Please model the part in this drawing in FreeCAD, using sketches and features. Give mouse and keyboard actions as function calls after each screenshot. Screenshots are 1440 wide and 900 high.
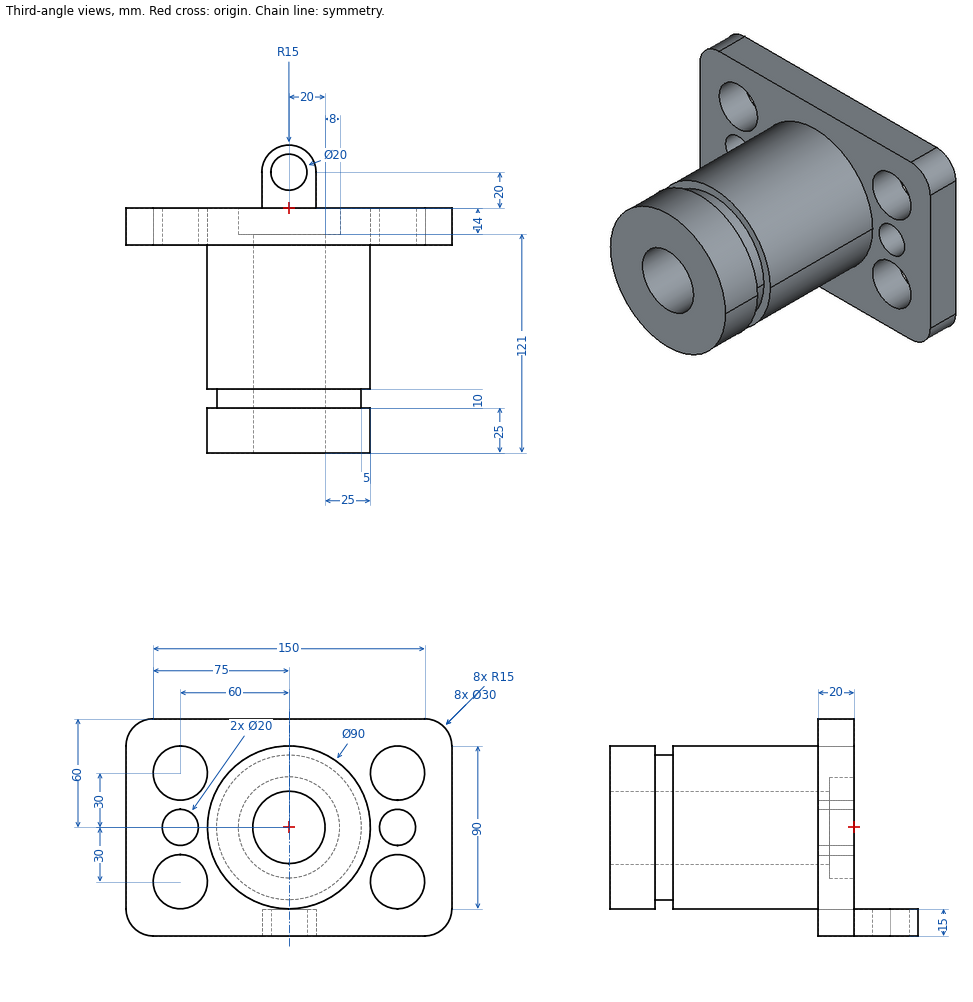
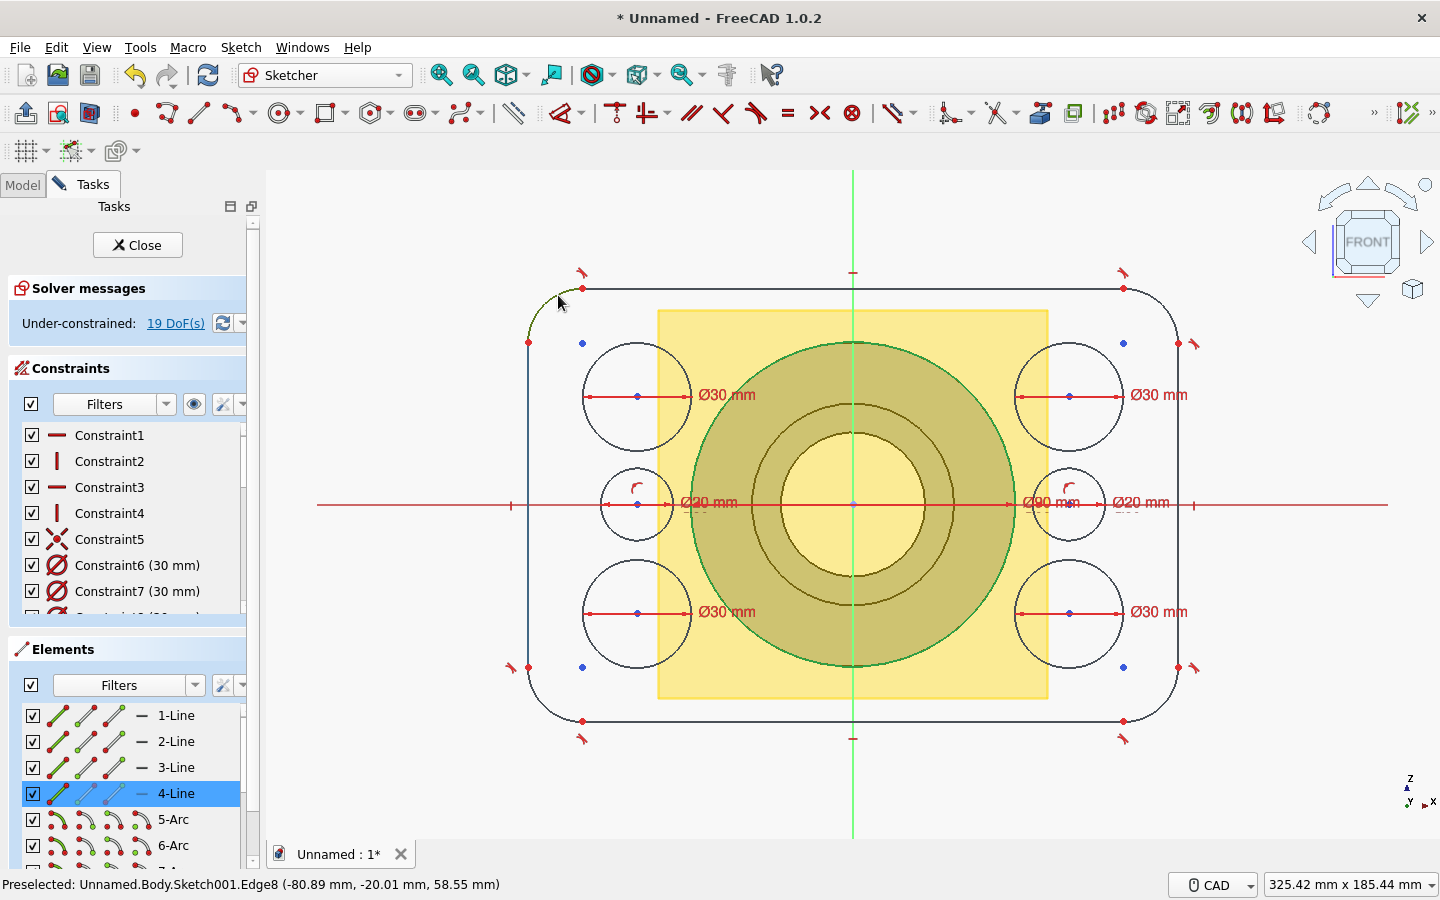
click(756, 114)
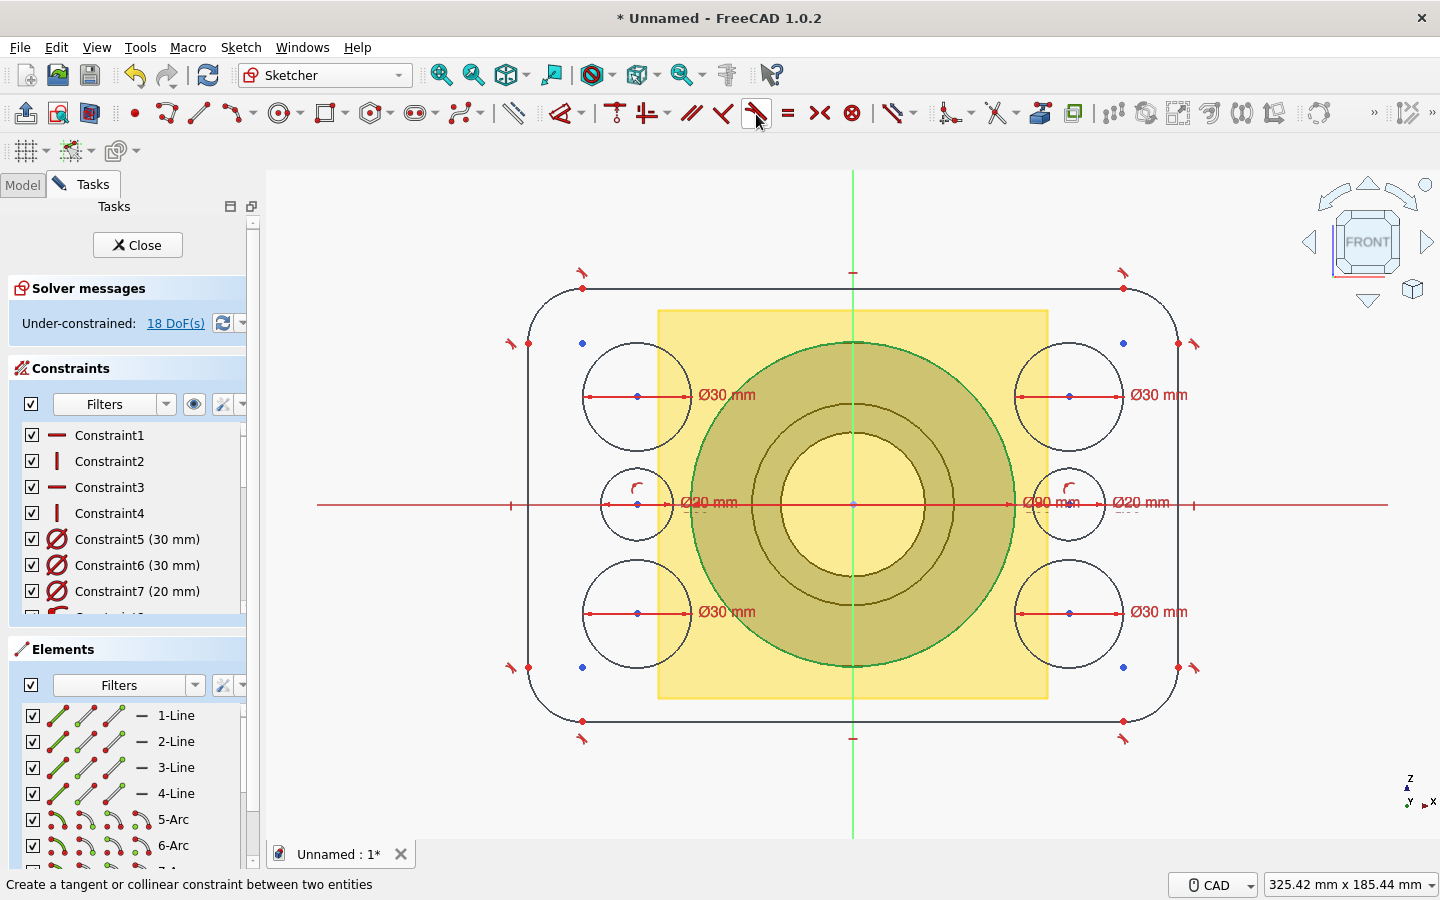
click(1172, 319)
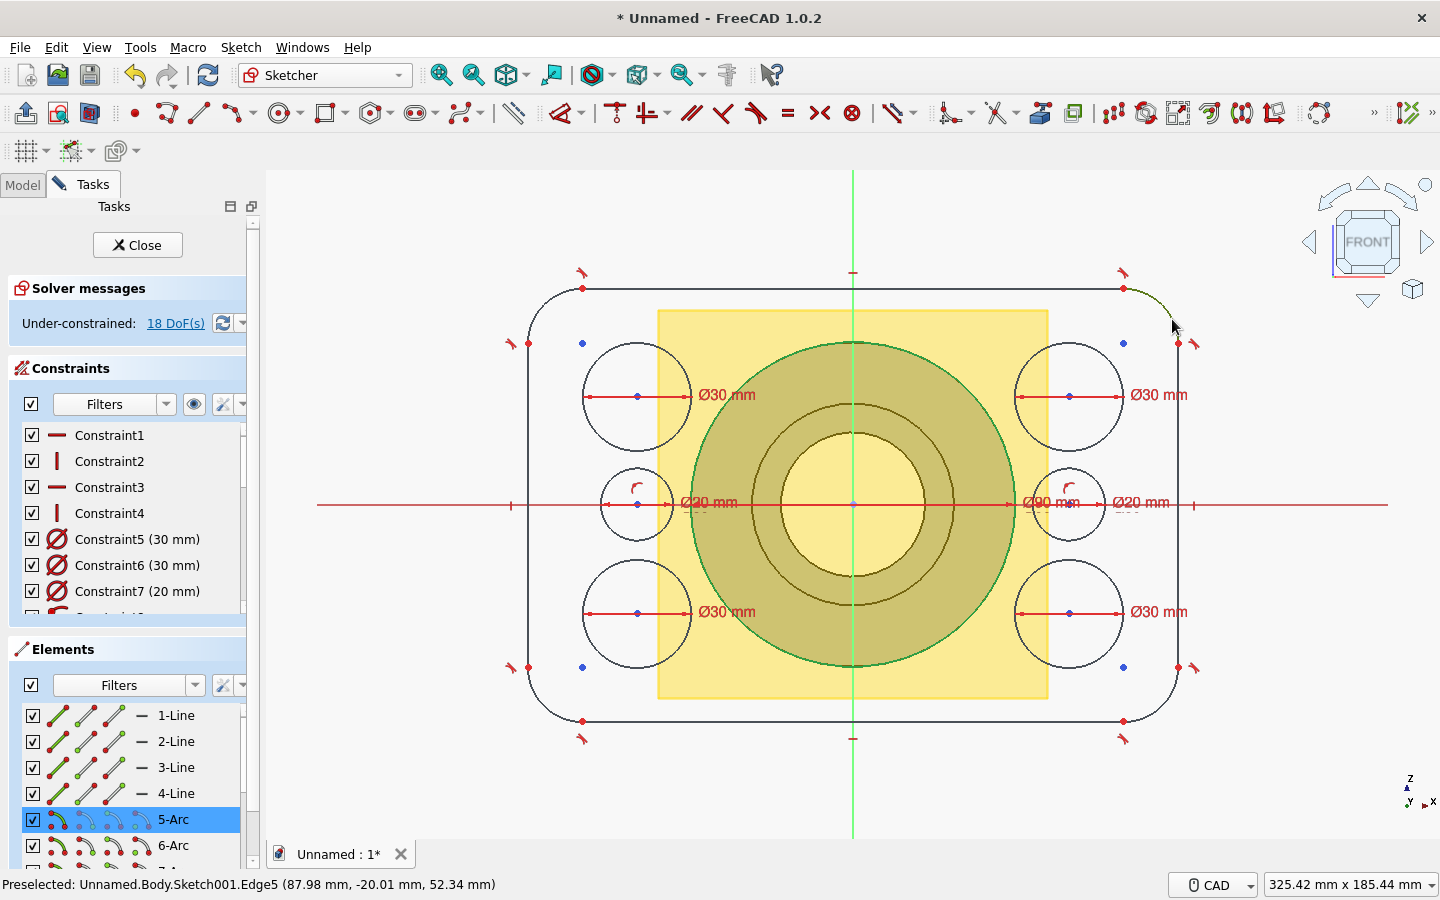
click(1148, 716)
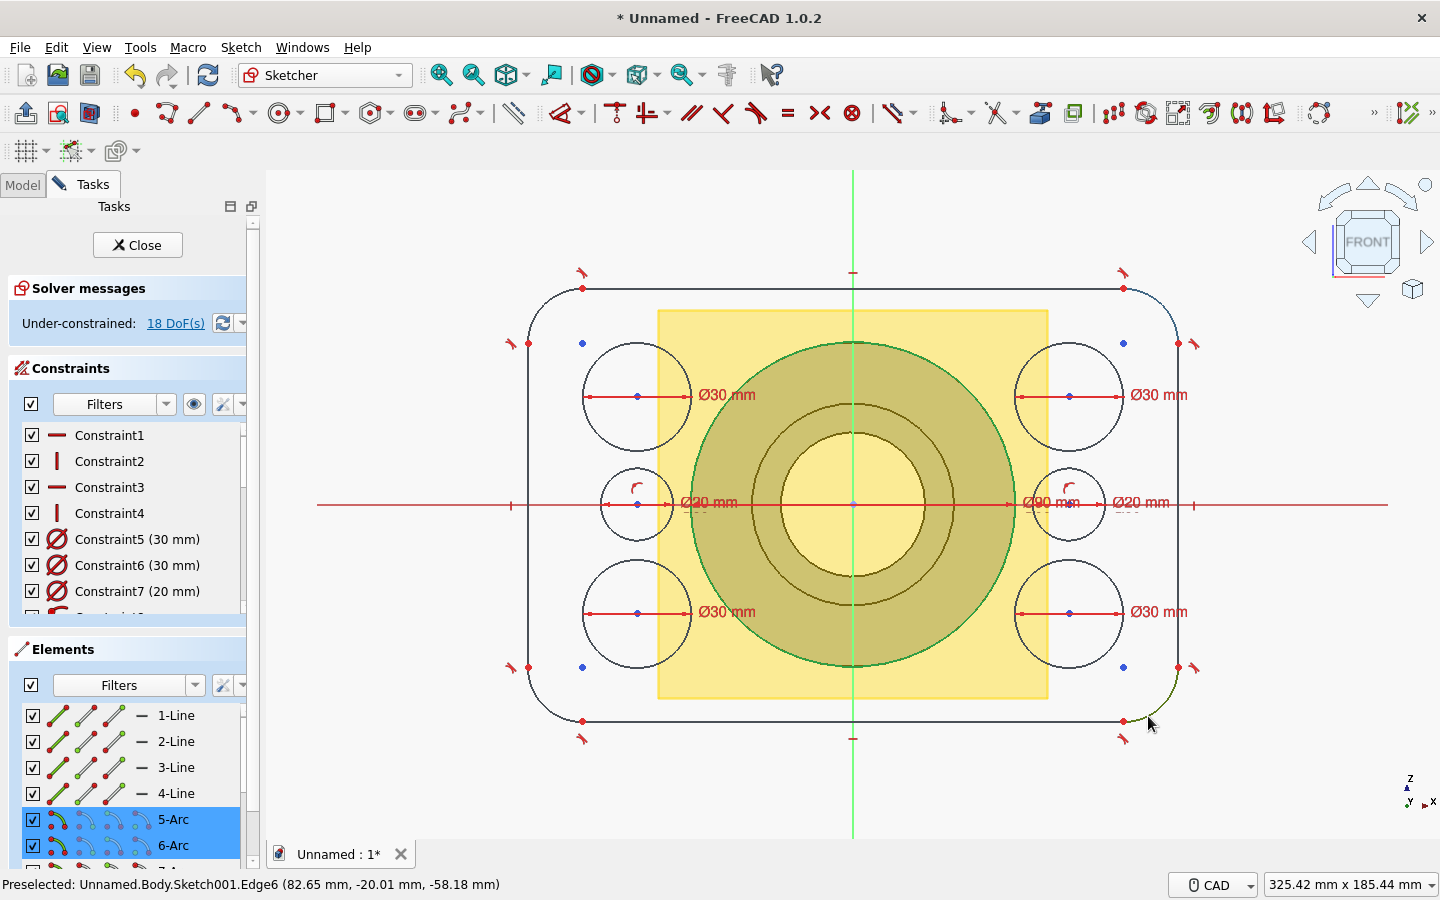
click(534, 692)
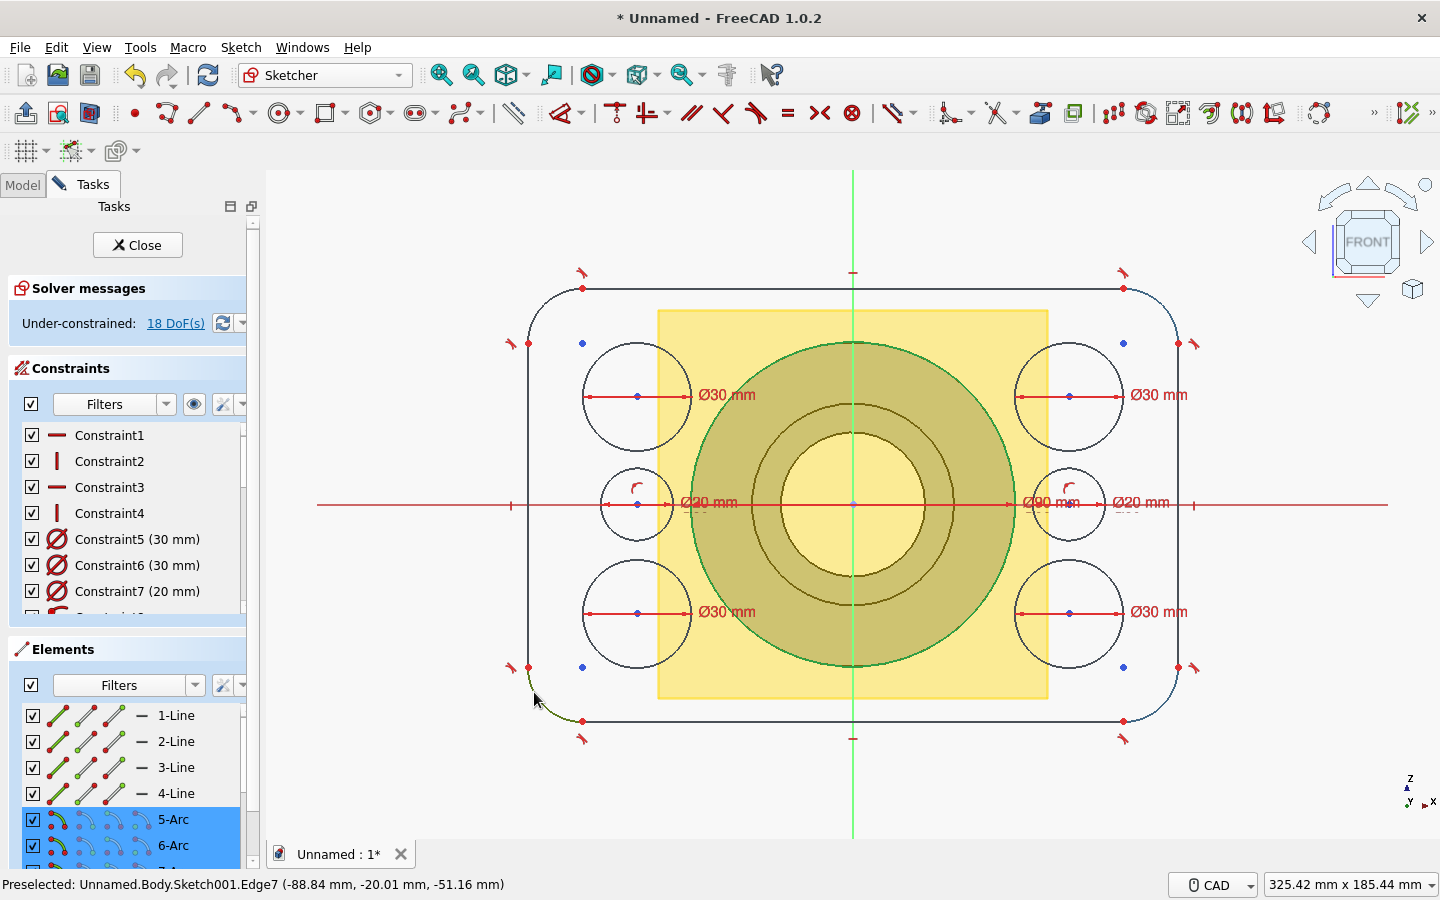
click(558, 295)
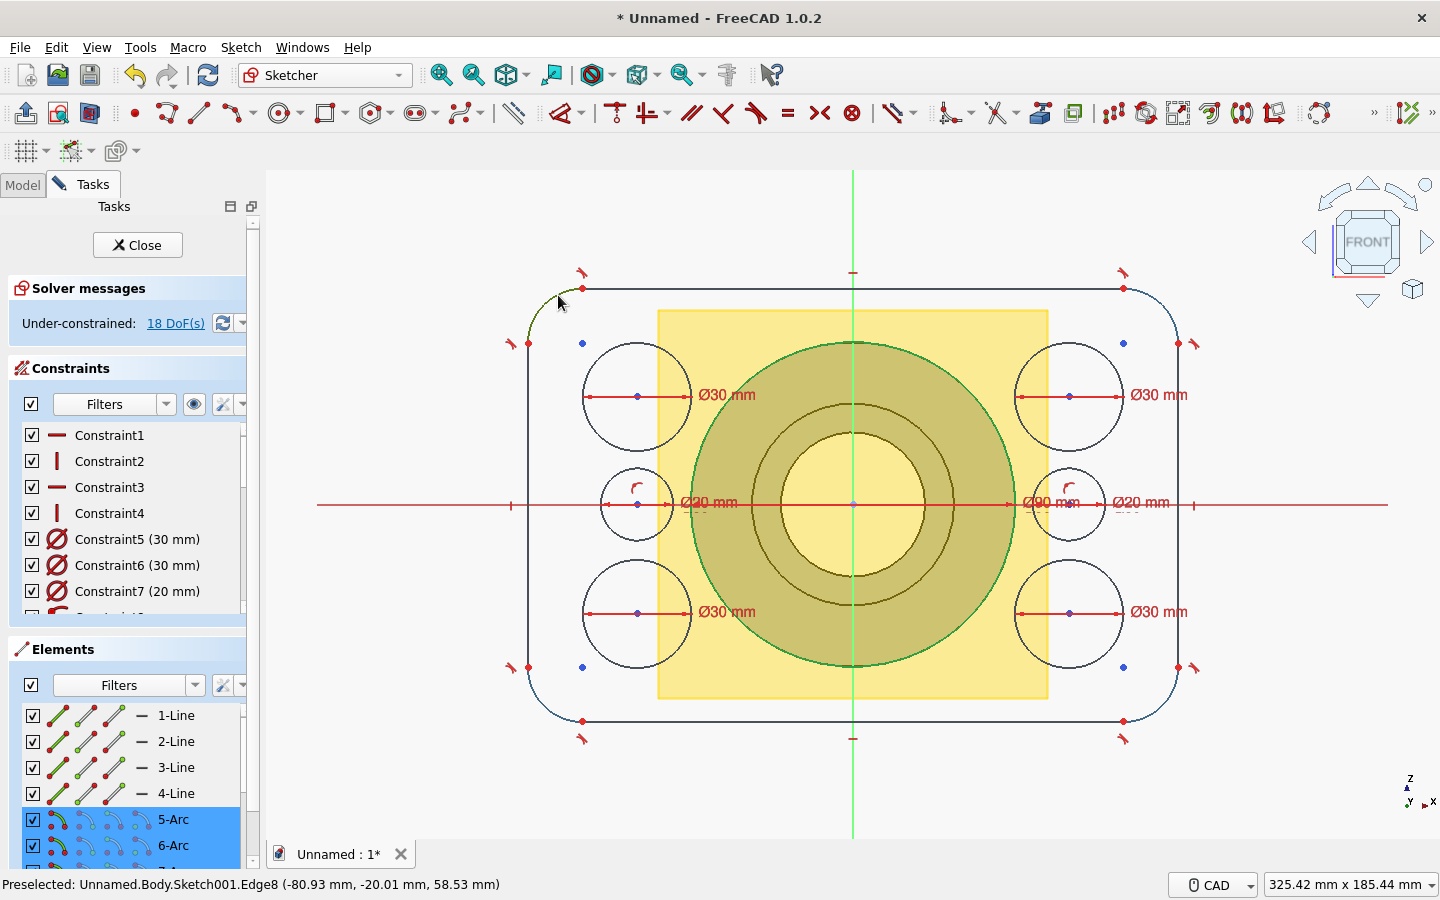
click(788, 114)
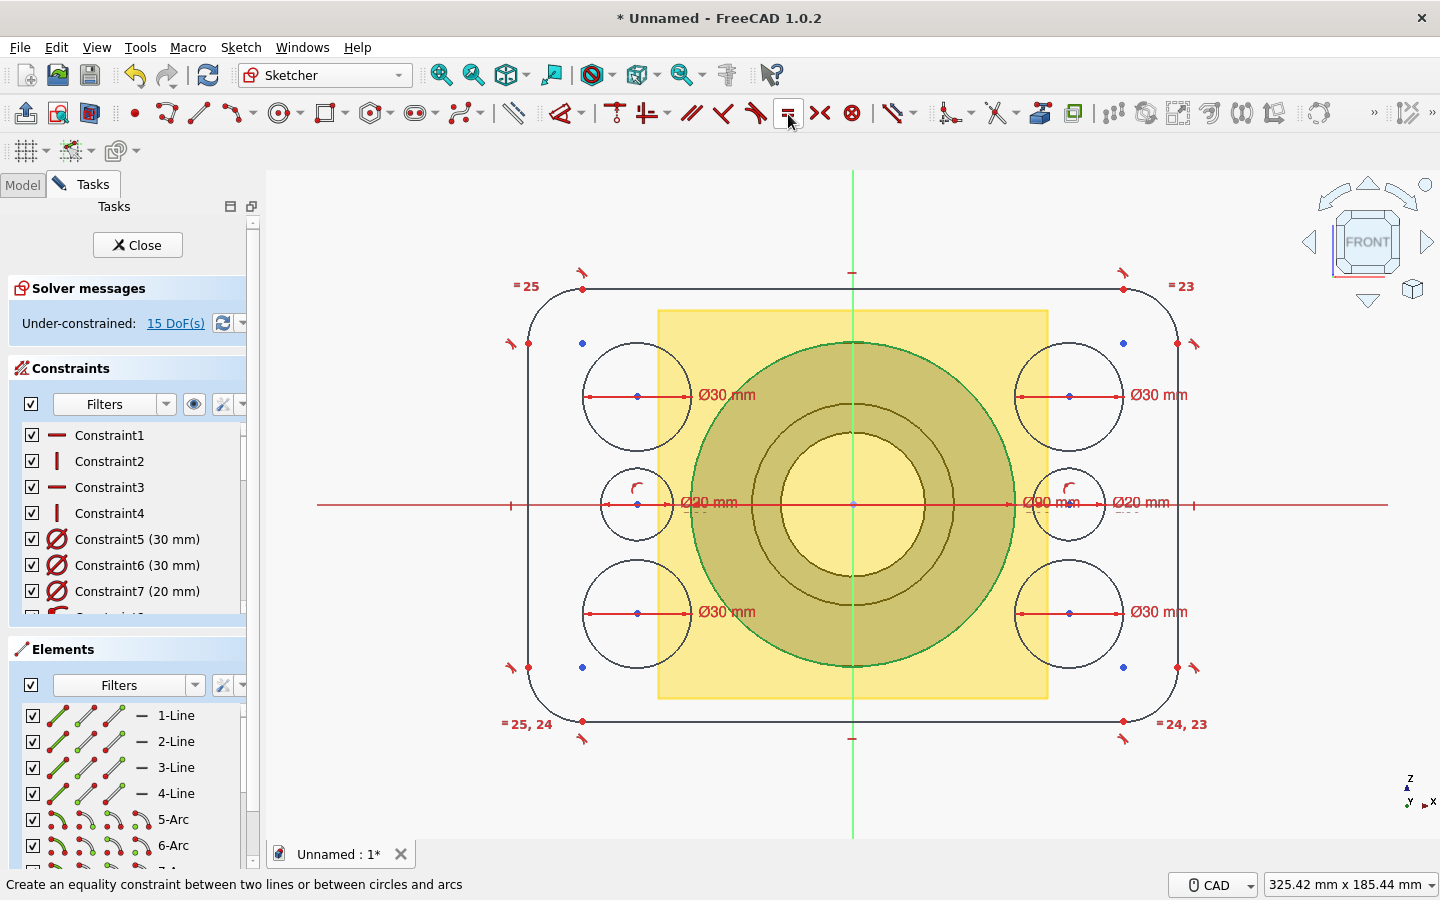
click(637, 397)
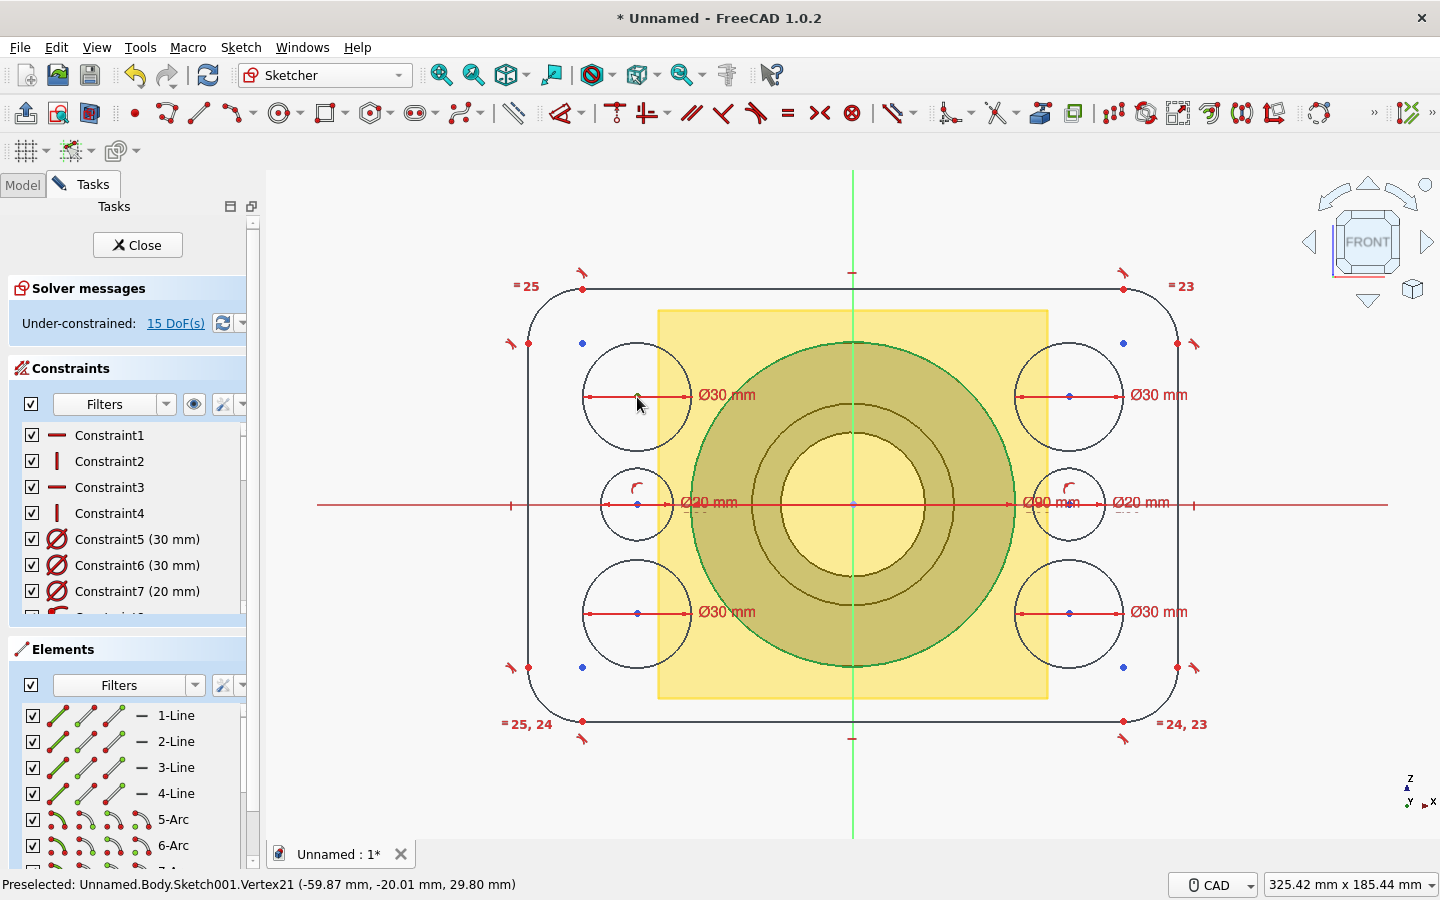
click(637, 504)